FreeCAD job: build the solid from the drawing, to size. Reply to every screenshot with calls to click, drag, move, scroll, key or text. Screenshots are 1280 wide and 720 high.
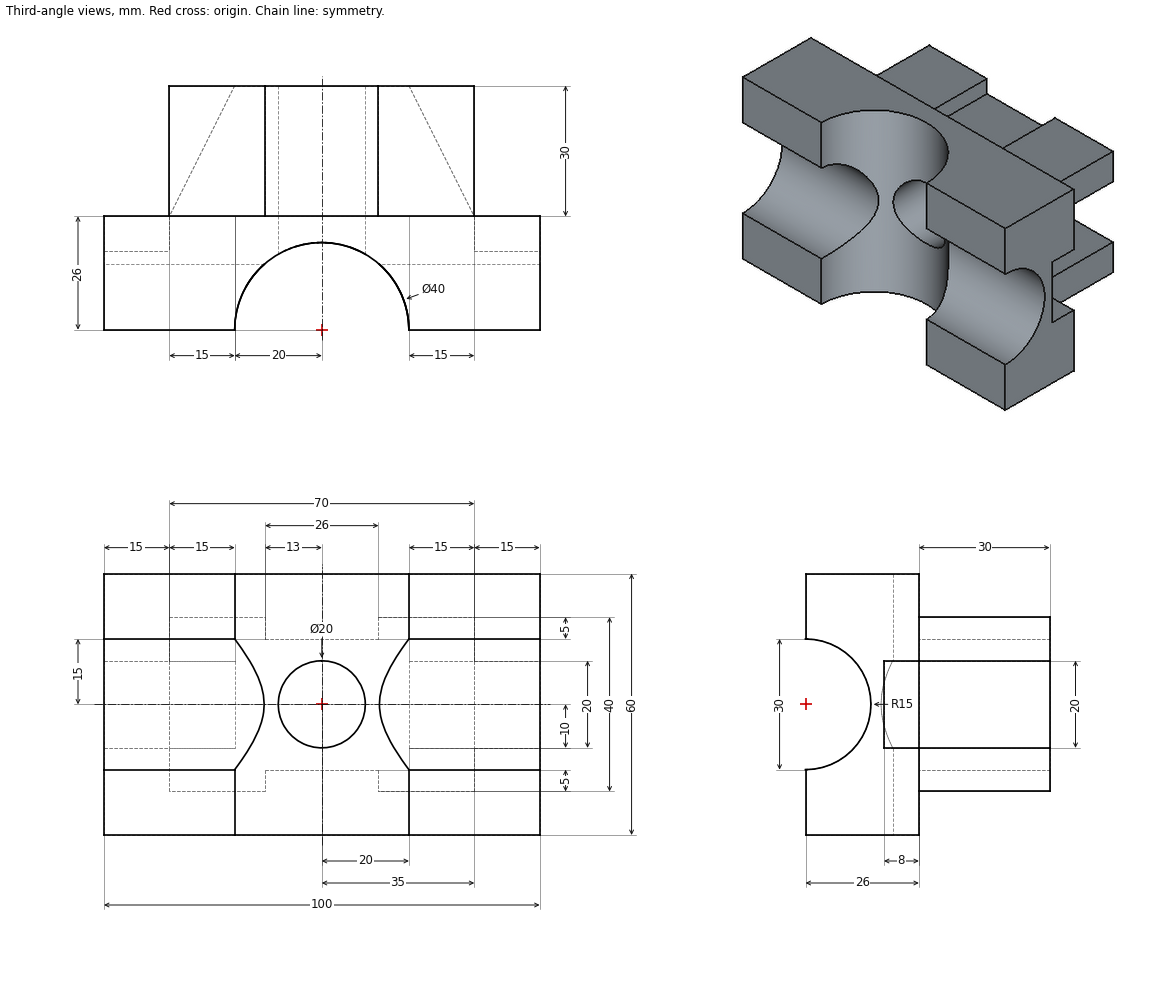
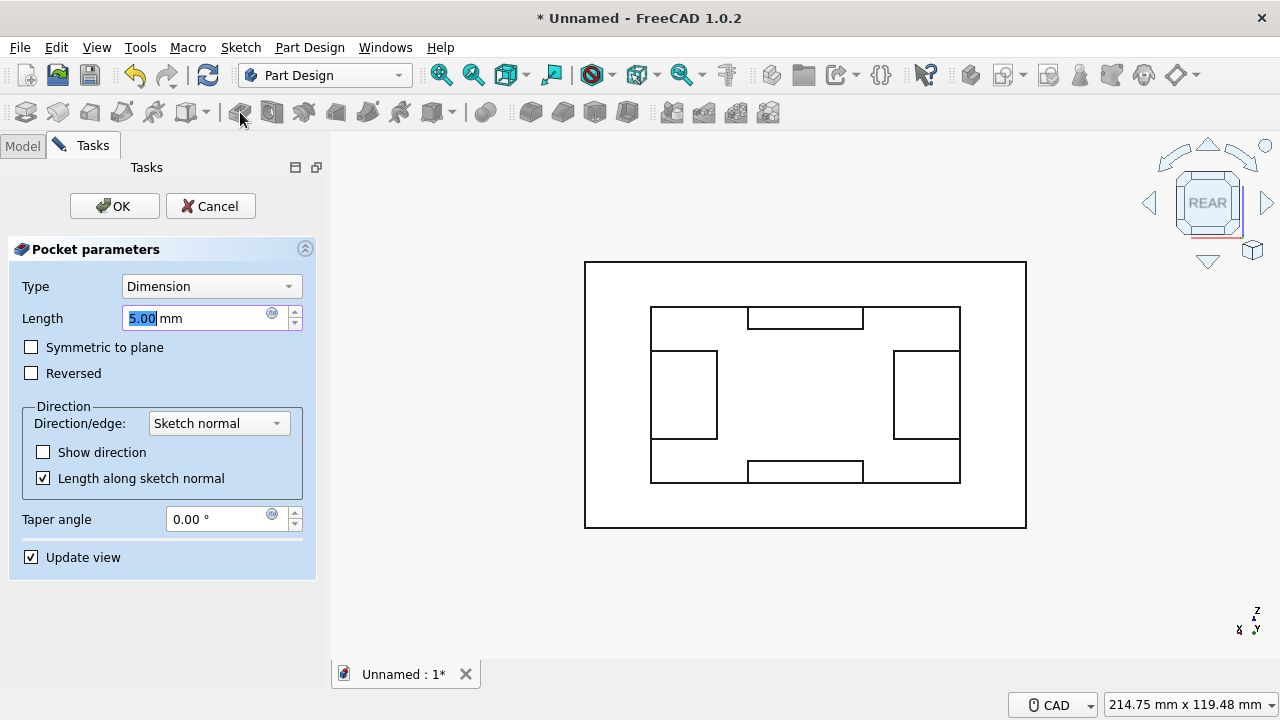
text(30)
key(Tab)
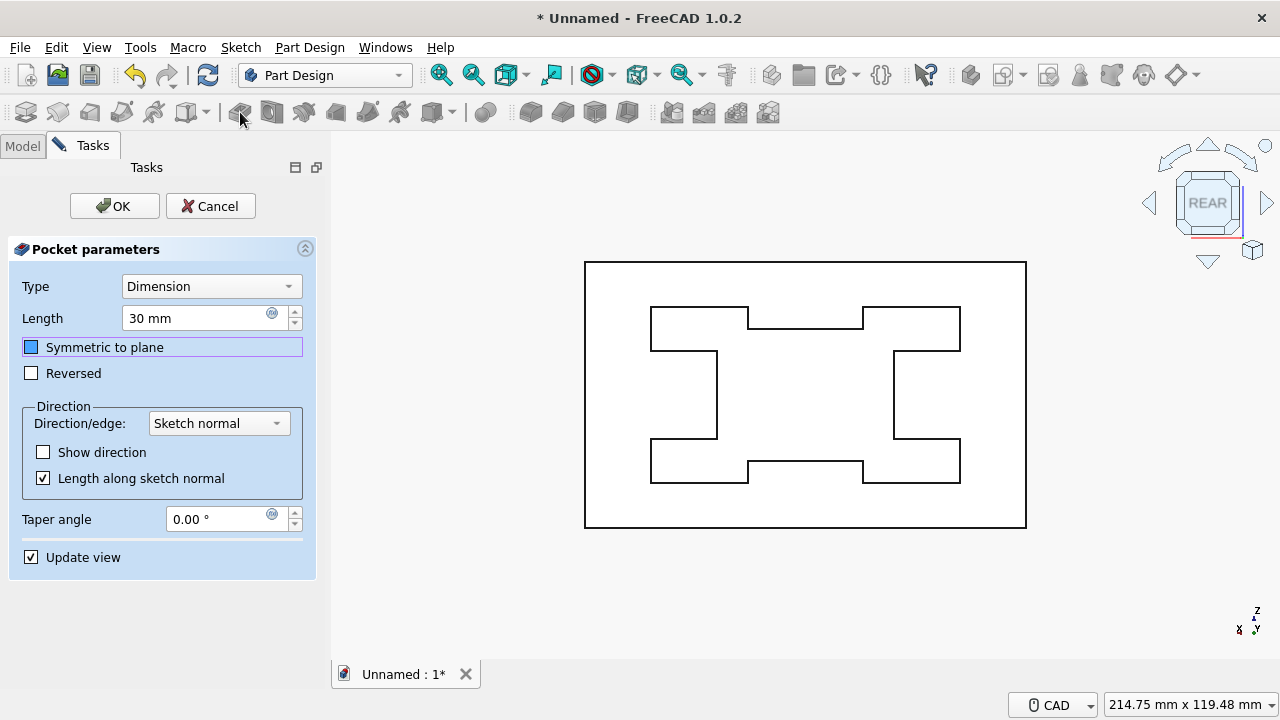
click(115, 206)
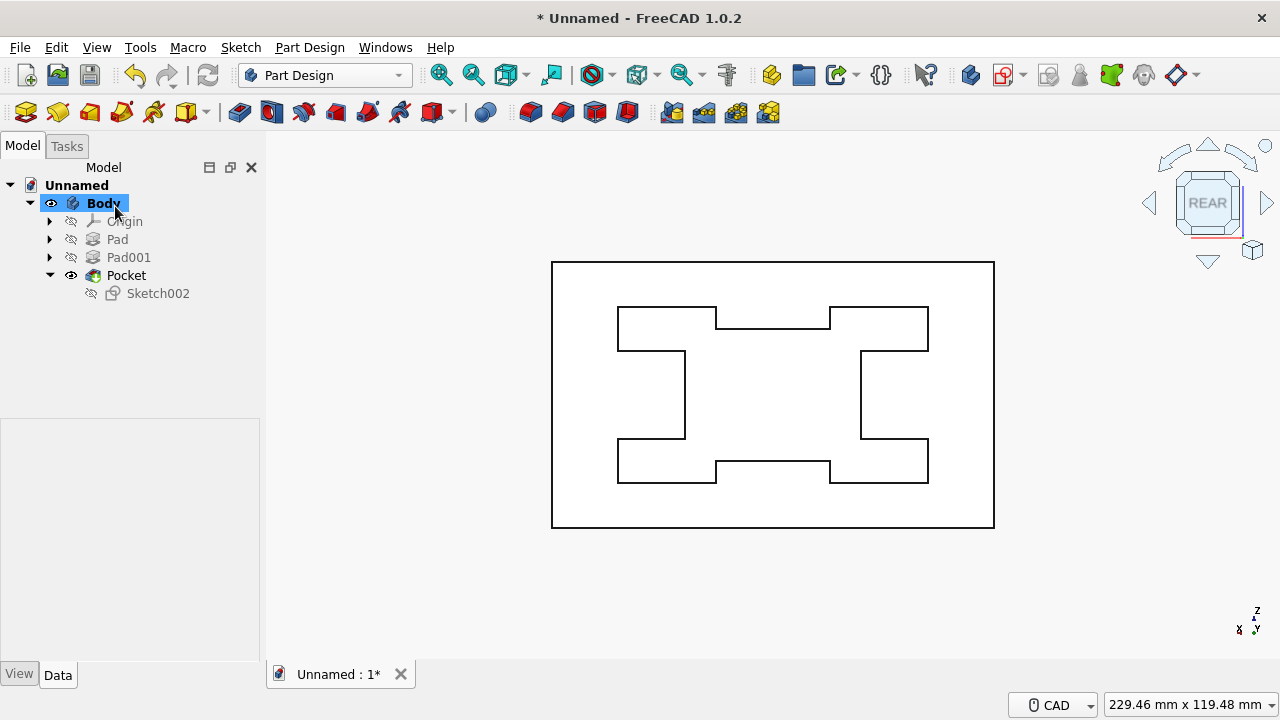
click(50, 221)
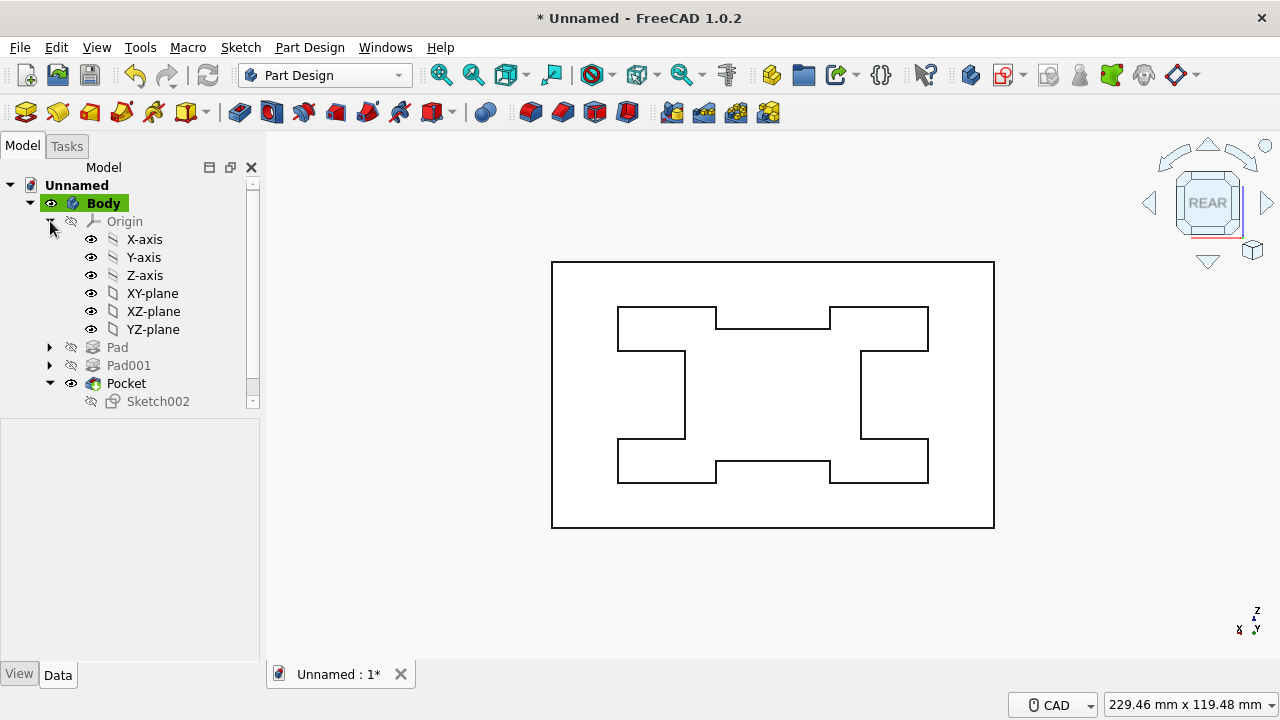
click(136, 293)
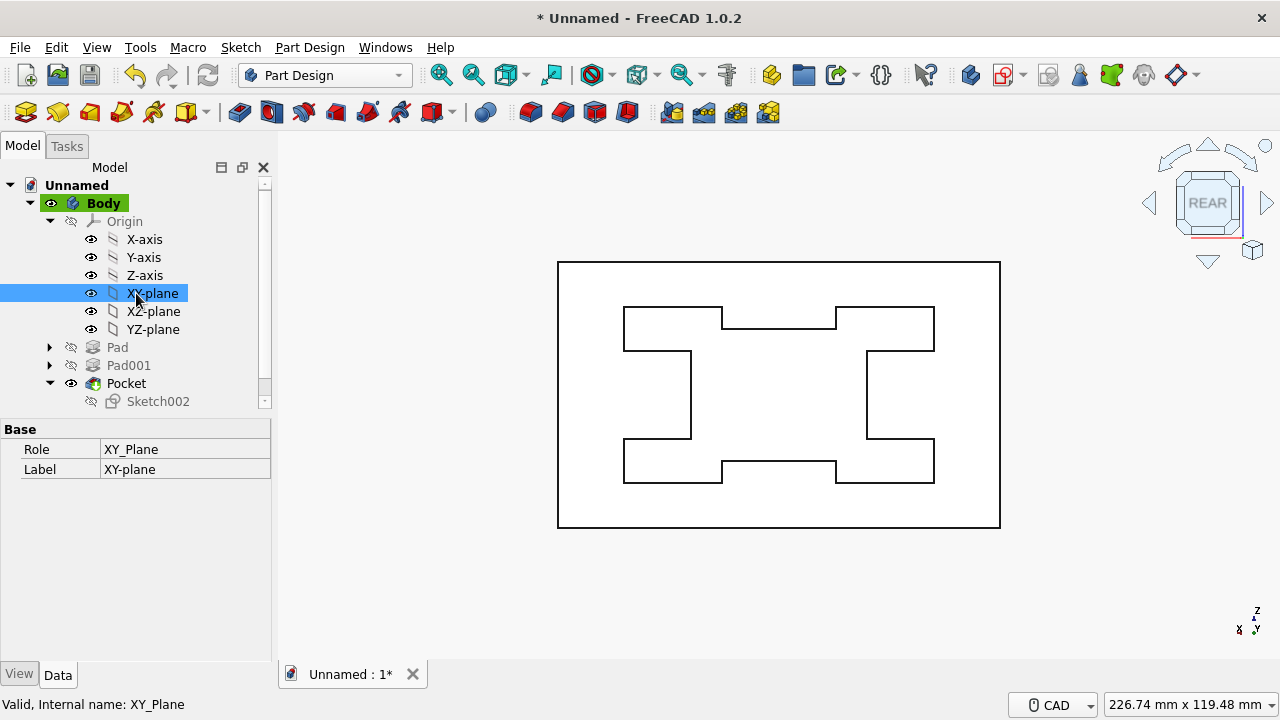
click(1176, 76)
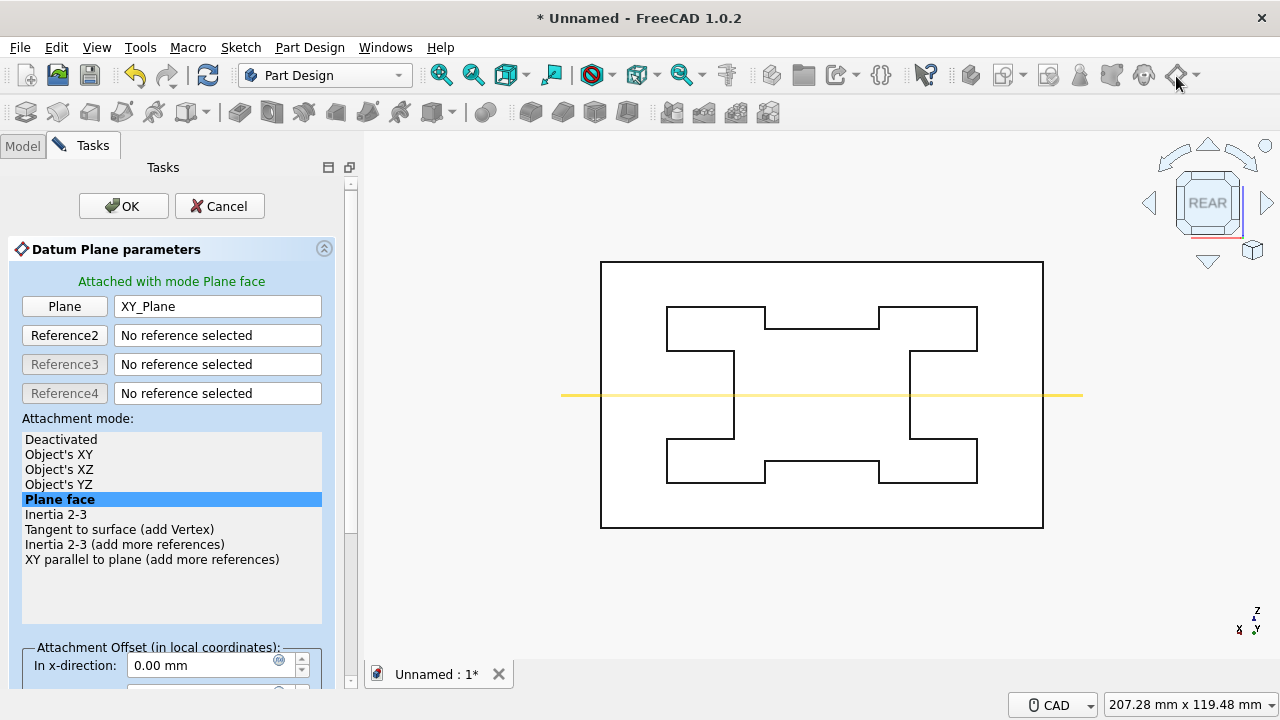
scroll(351, 432, down, 2)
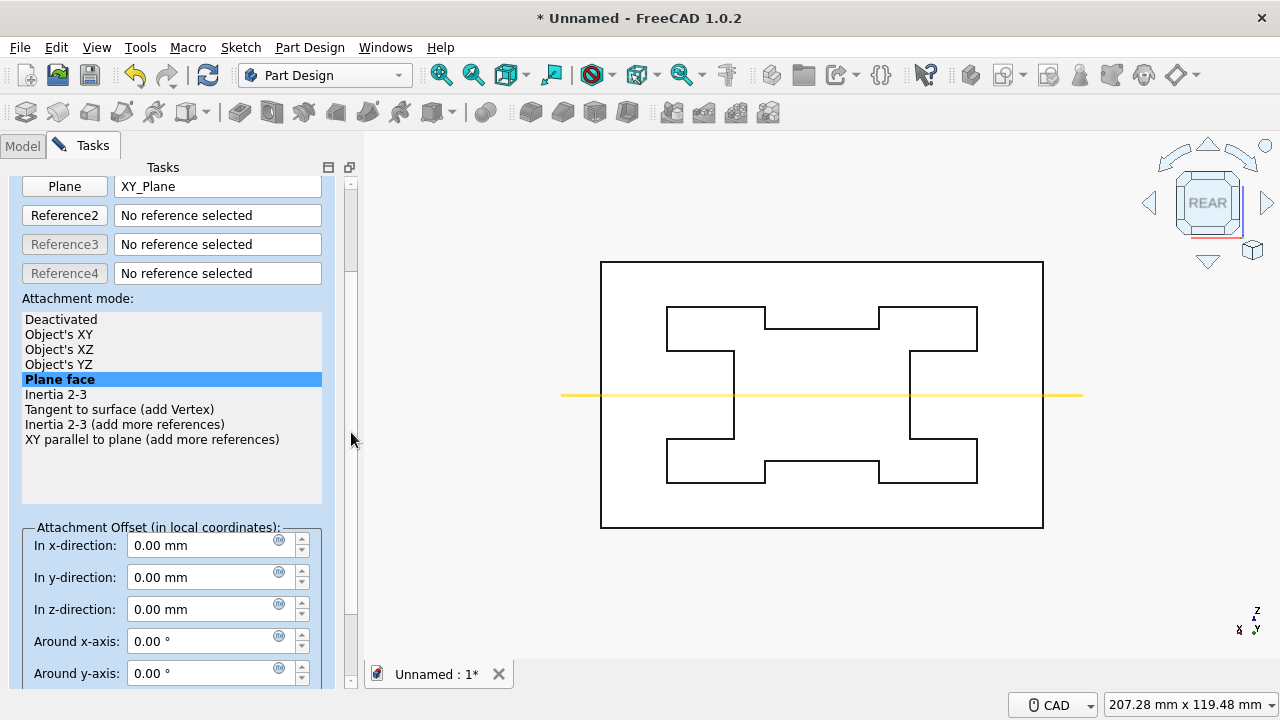
triple_click(210, 609)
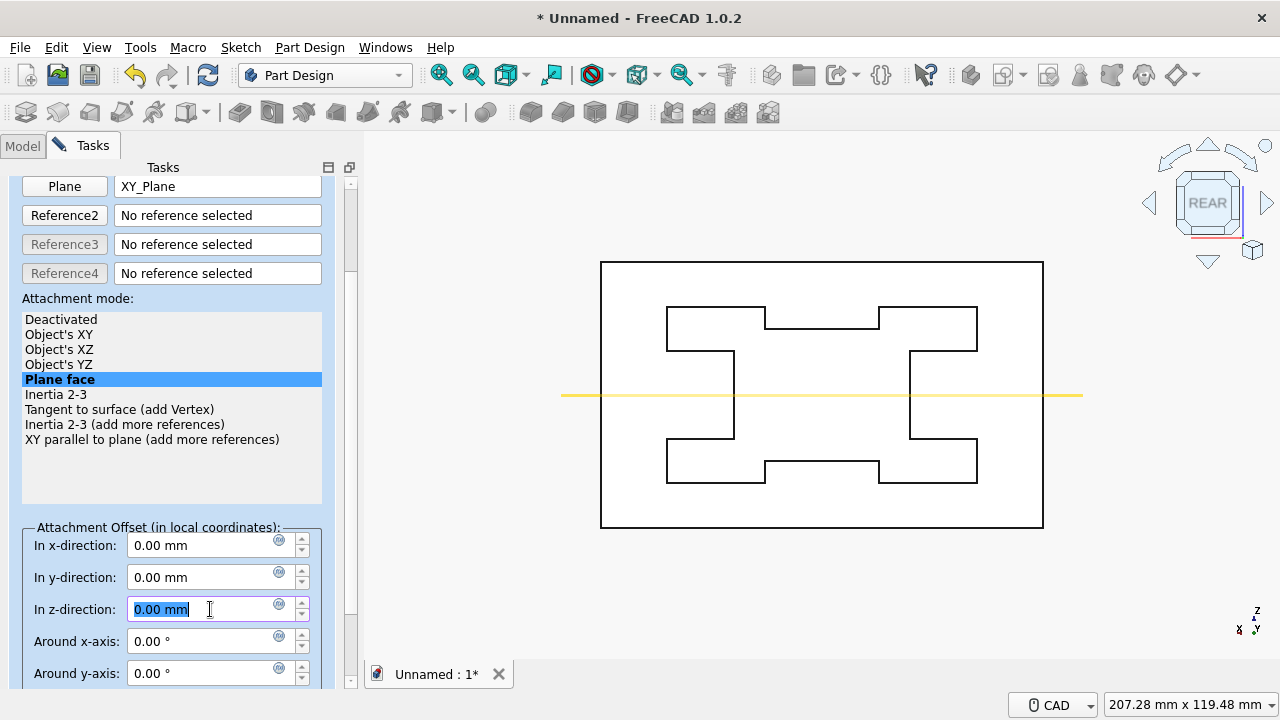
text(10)
key(Tab)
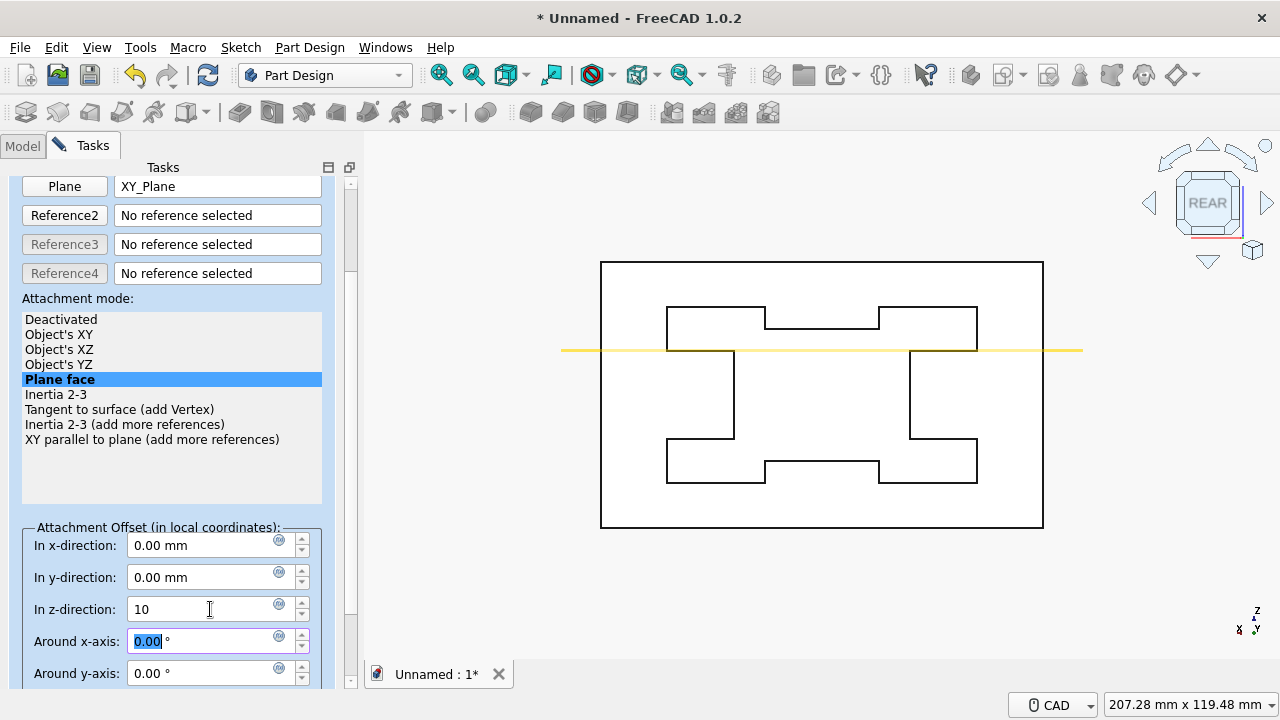
scroll(351, 432, up, 3)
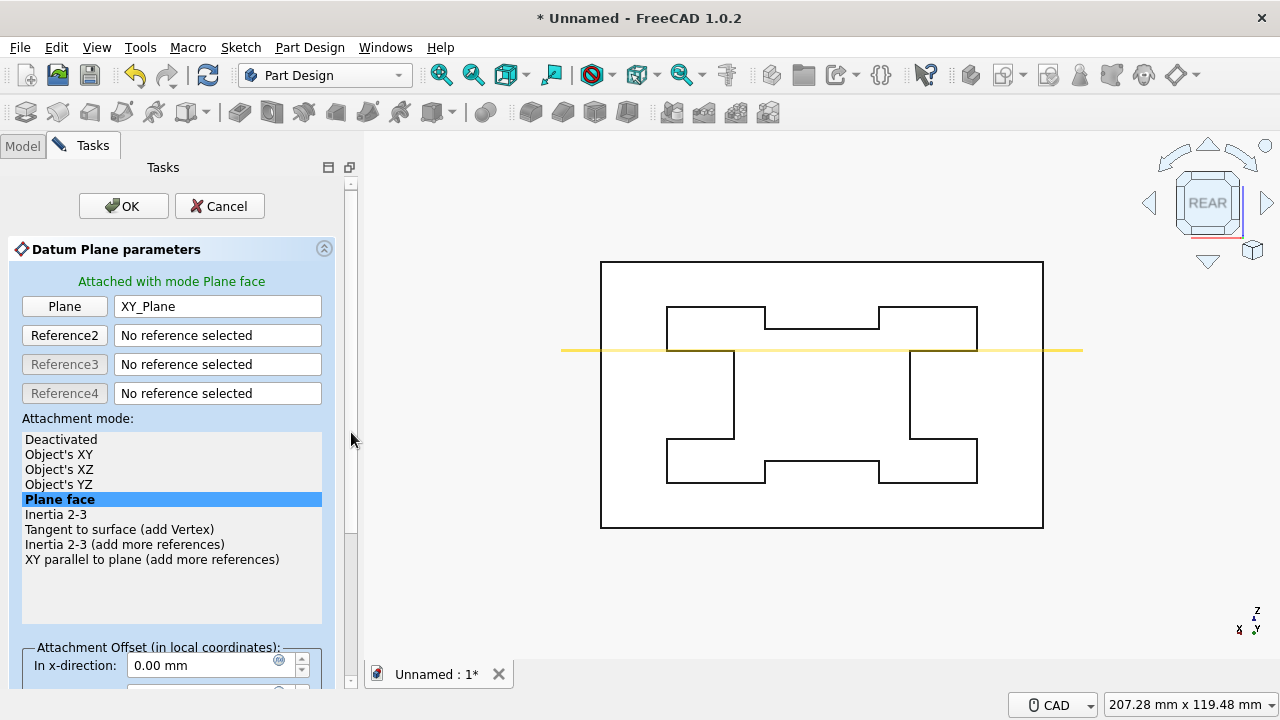
click(124, 206)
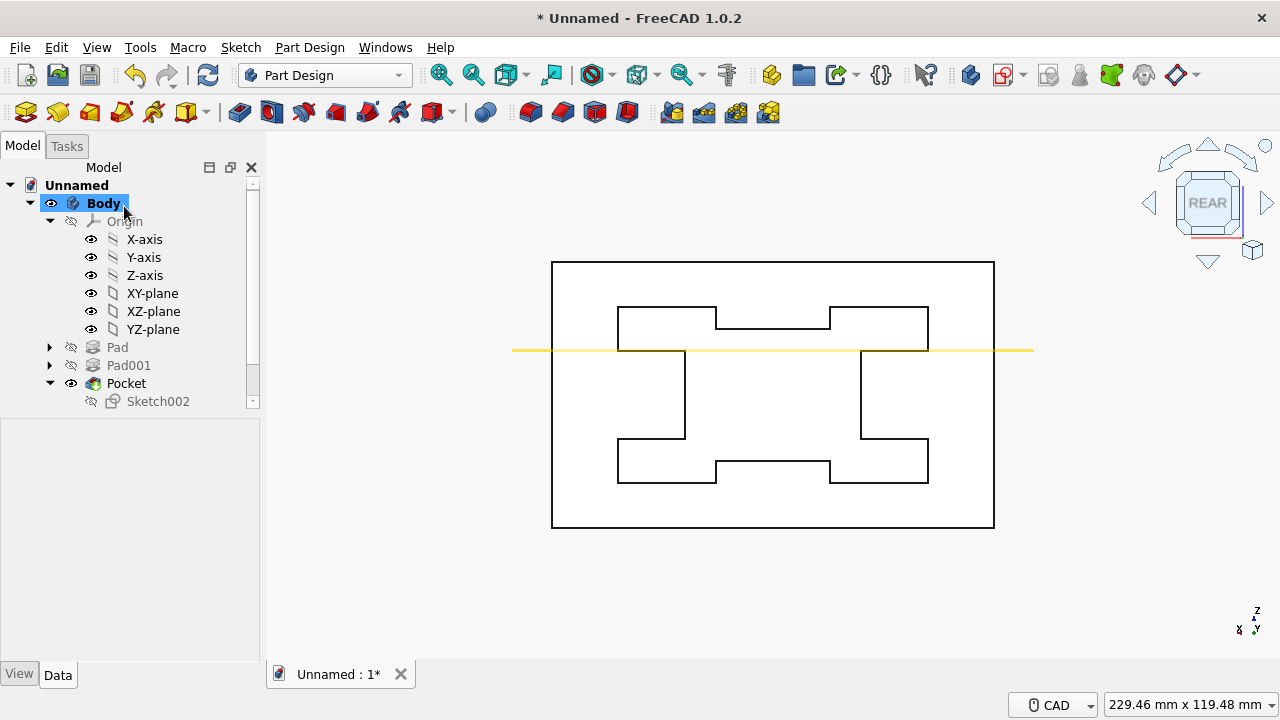
scroll(100, 289, down, 3)